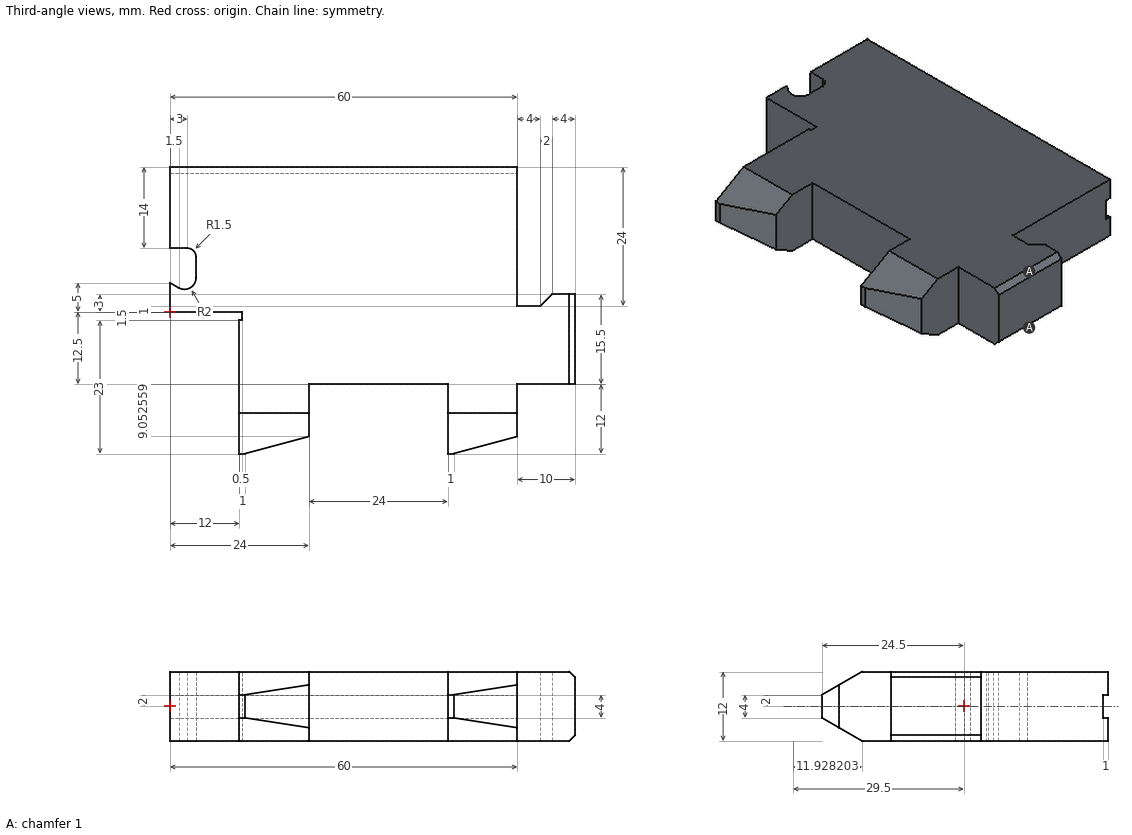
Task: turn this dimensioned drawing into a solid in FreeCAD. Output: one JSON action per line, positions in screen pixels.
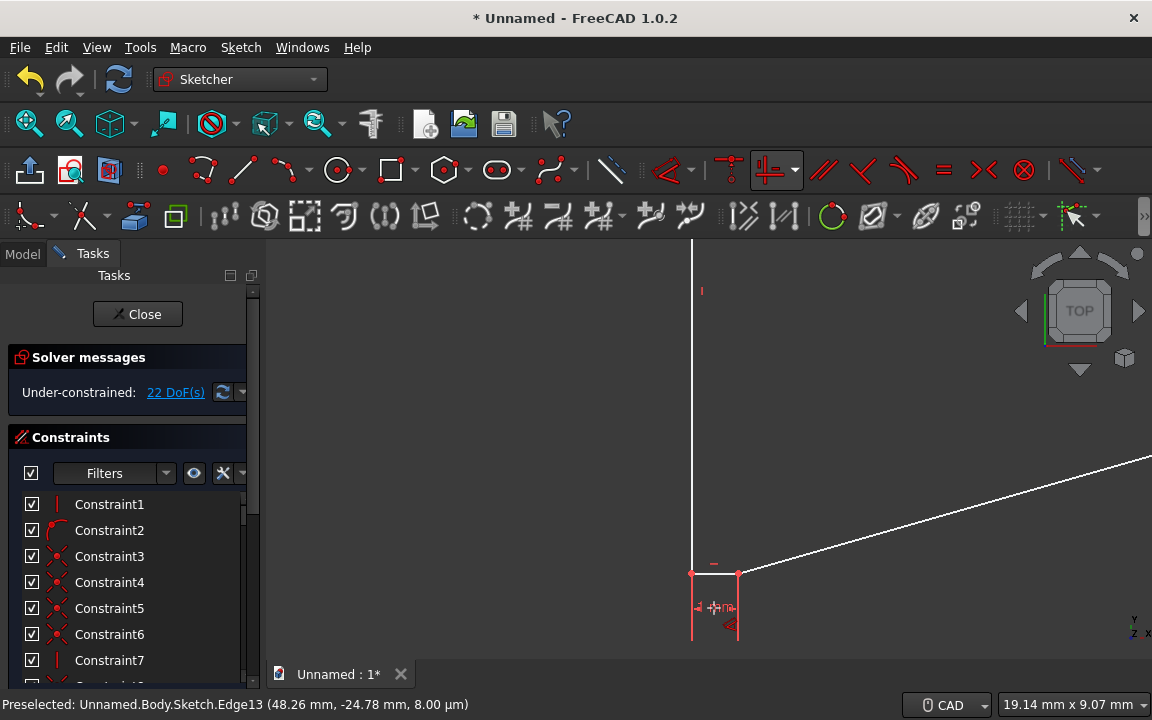
{"action": "scroll", "coordinate": [709, 578], "scroll_direction": "down", "scroll_amount": 11}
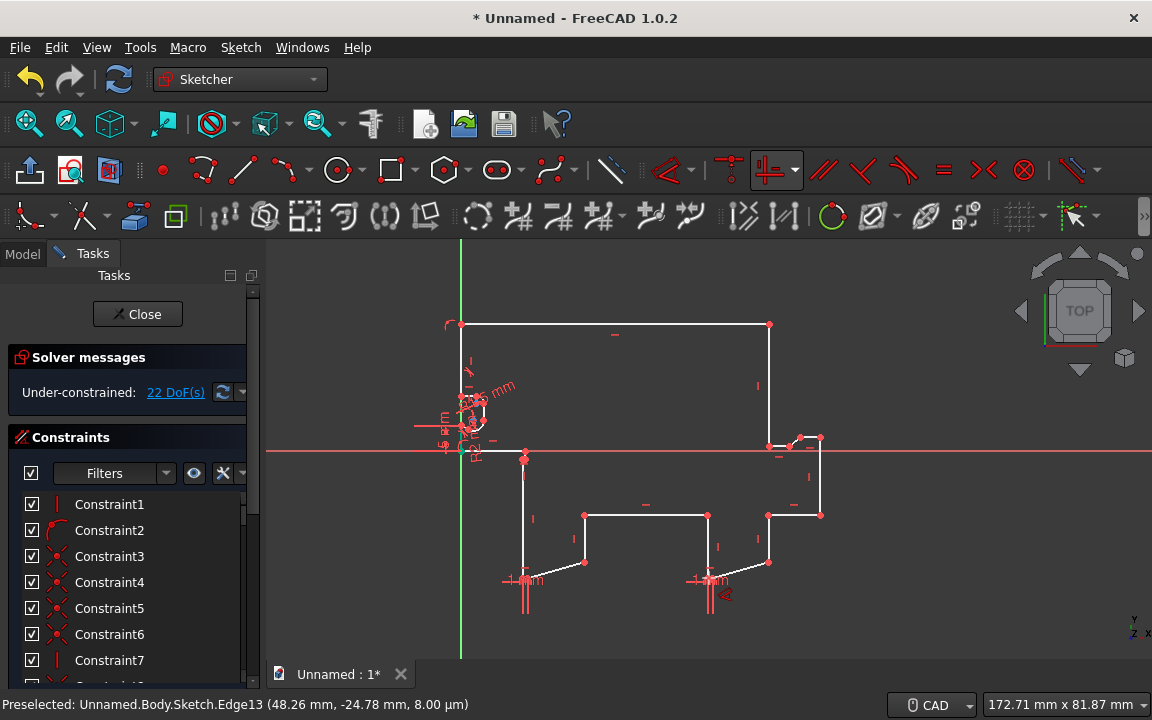
{"action": "scroll", "coordinate": [814, 437], "scroll_direction": "up", "scroll_amount": 5}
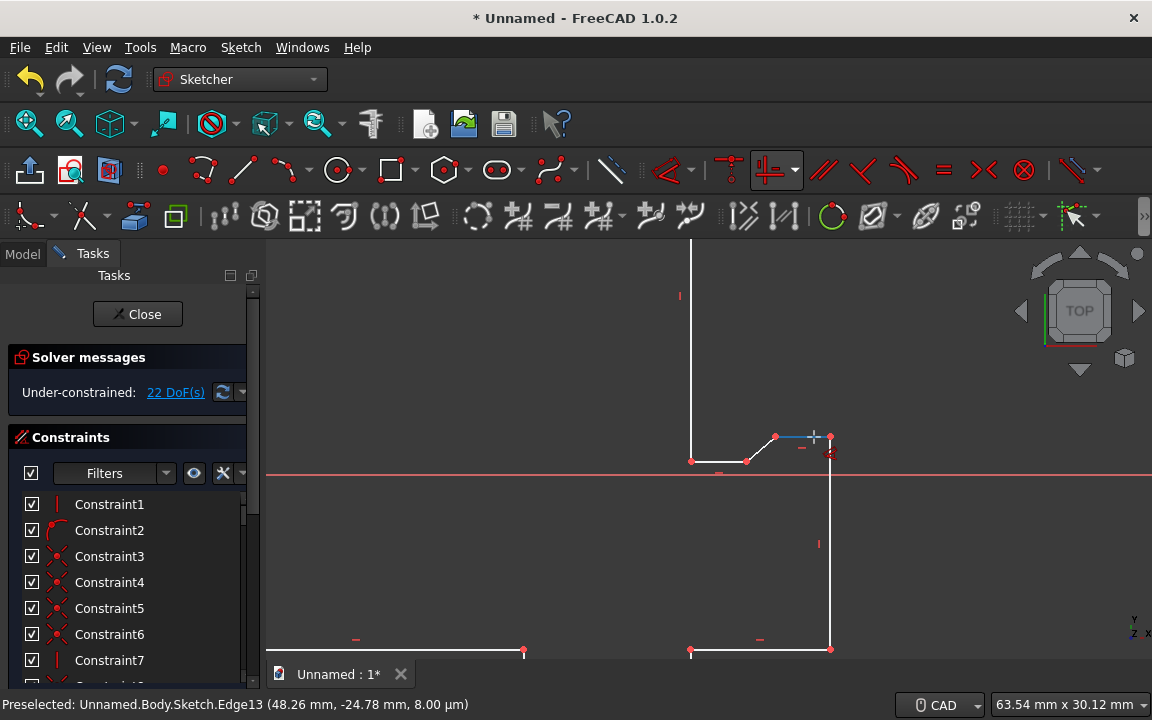
{"action": "left_click", "coordinate": [814, 437]}
{"action": "left_click", "coordinate": [803, 403]}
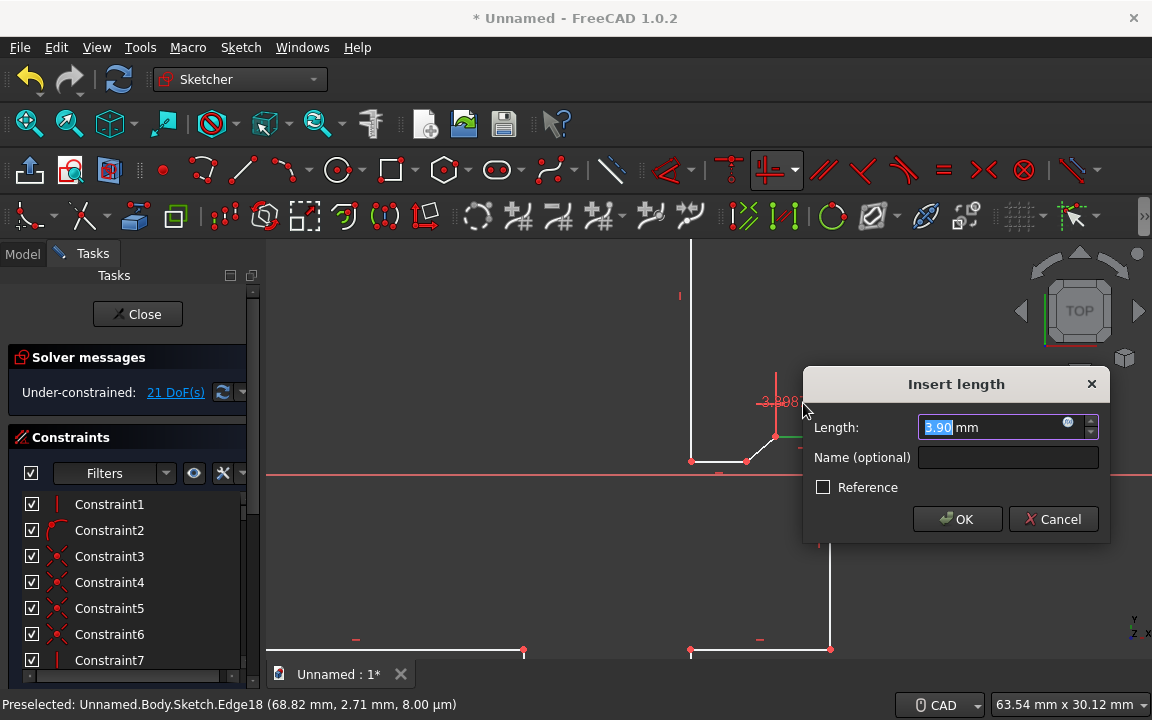
{"action": "type", "text": "4"}
{"action": "key", "text": "Return"}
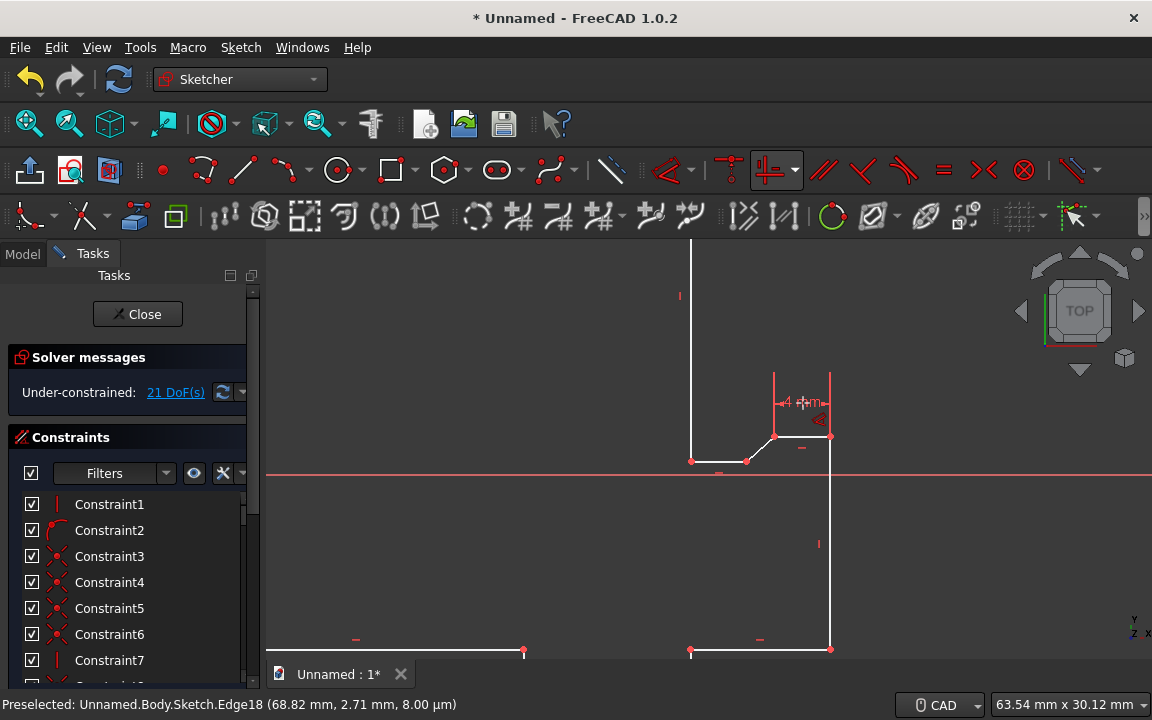
{"action": "left_click", "coordinate": [730, 462]}
{"action": "left_click", "coordinate": [719, 428]}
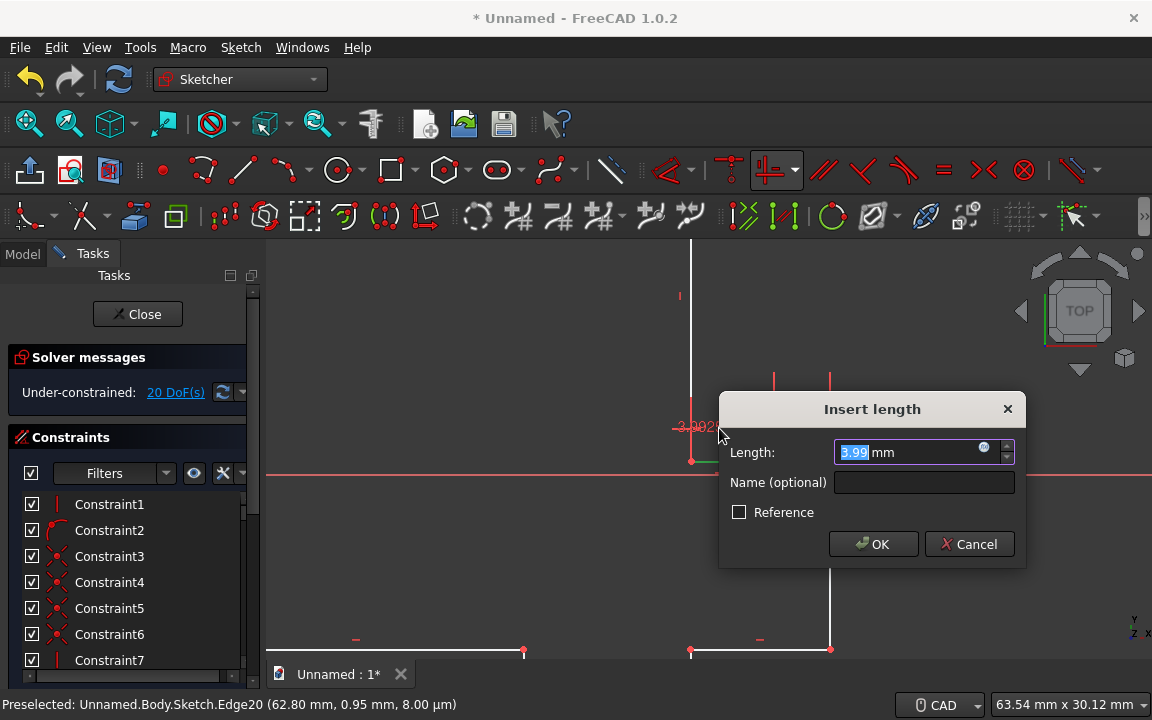
{"action": "type", "text": "4"}
{"action": "key", "text": "Return"}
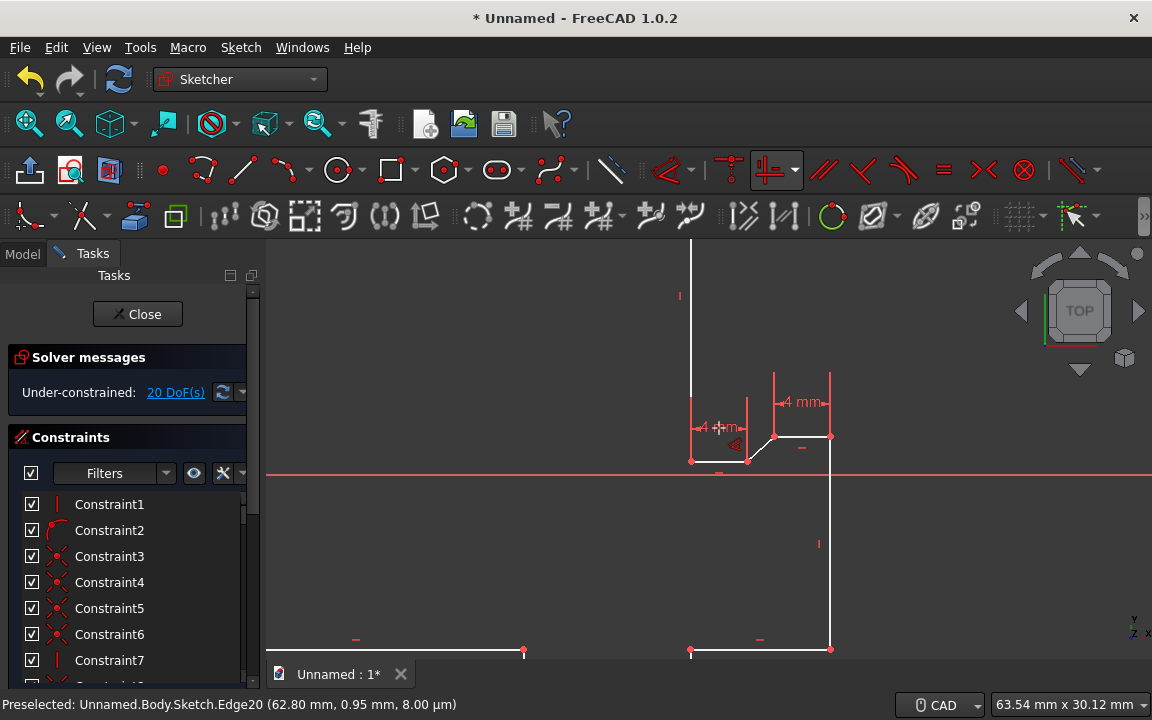
{"action": "scroll", "coordinate": [814, 436], "scroll_direction": "down", "scroll_amount": 5}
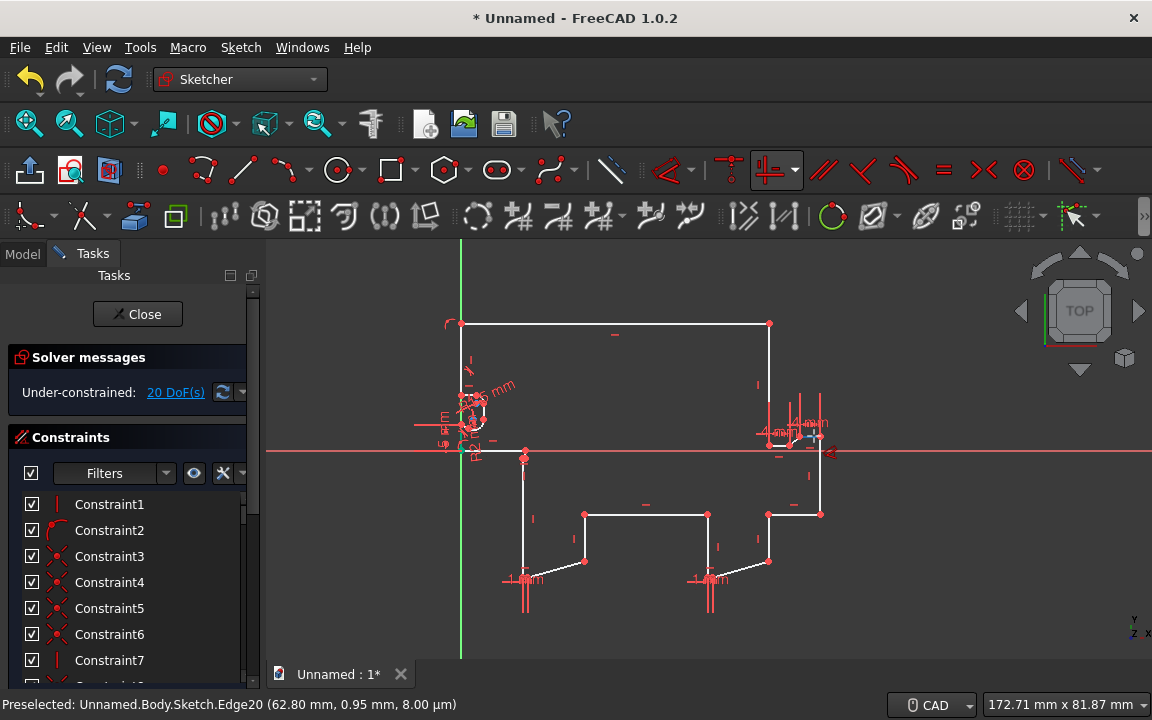
{"action": "scroll", "coordinate": [466, 395], "scroll_direction": "up", "scroll_amount": 6}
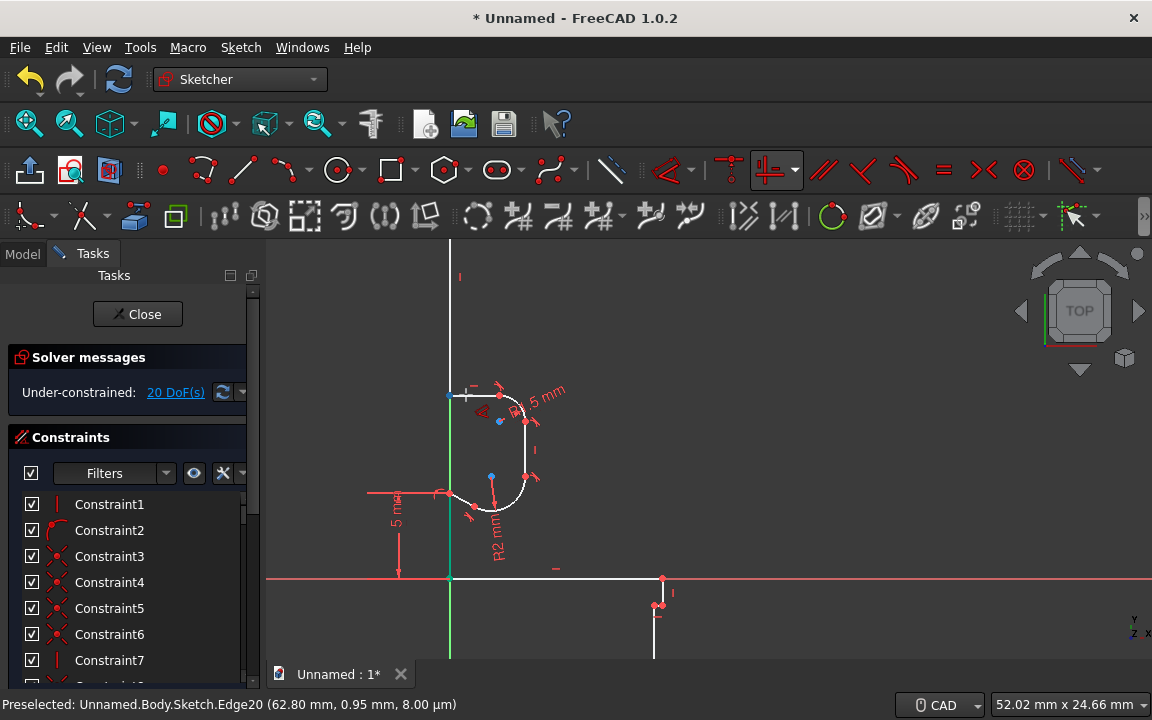
{"action": "left_click", "coordinate": [465, 396]}
{"action": "left_click", "coordinate": [475, 362]}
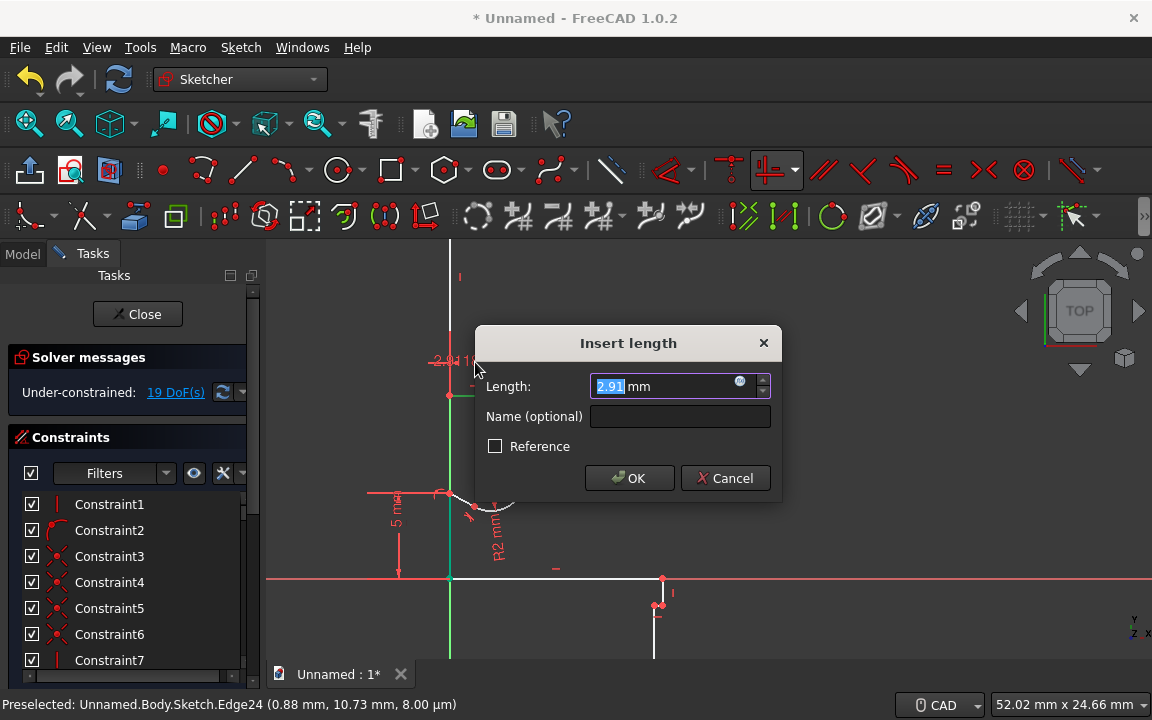
{"action": "type", "text": "3"}
{"action": "key", "text": "Return"}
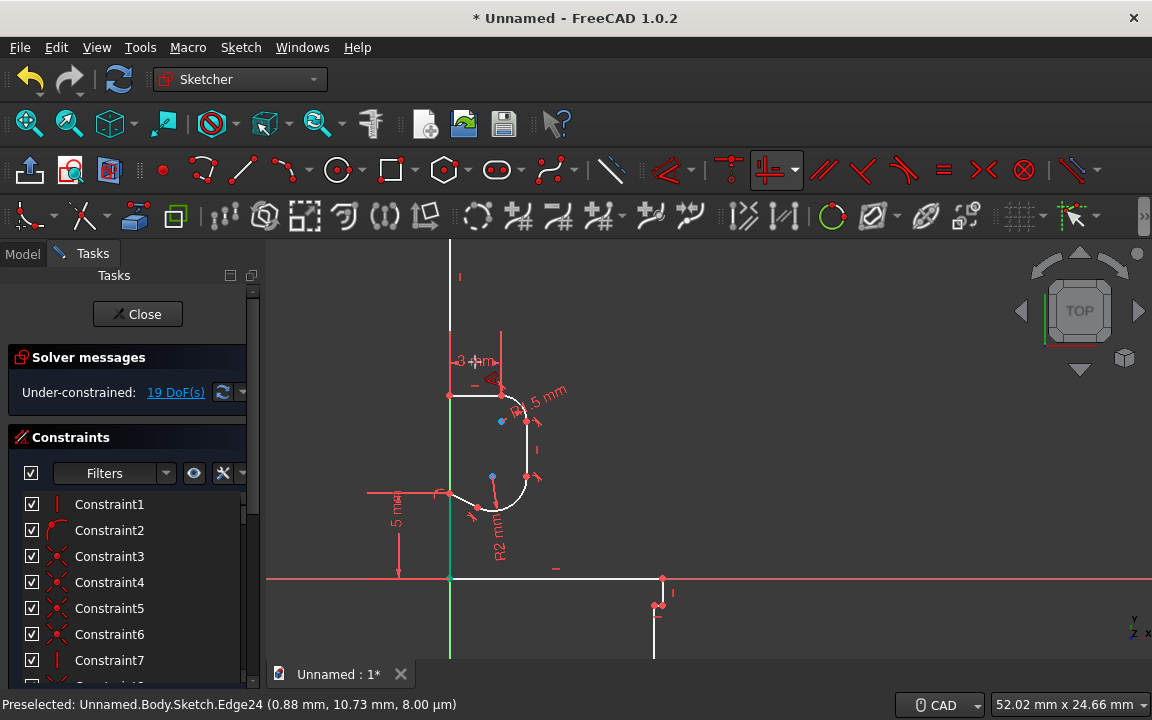
{"action": "scroll", "coordinate": [466, 395], "scroll_direction": "down", "scroll_amount": 6}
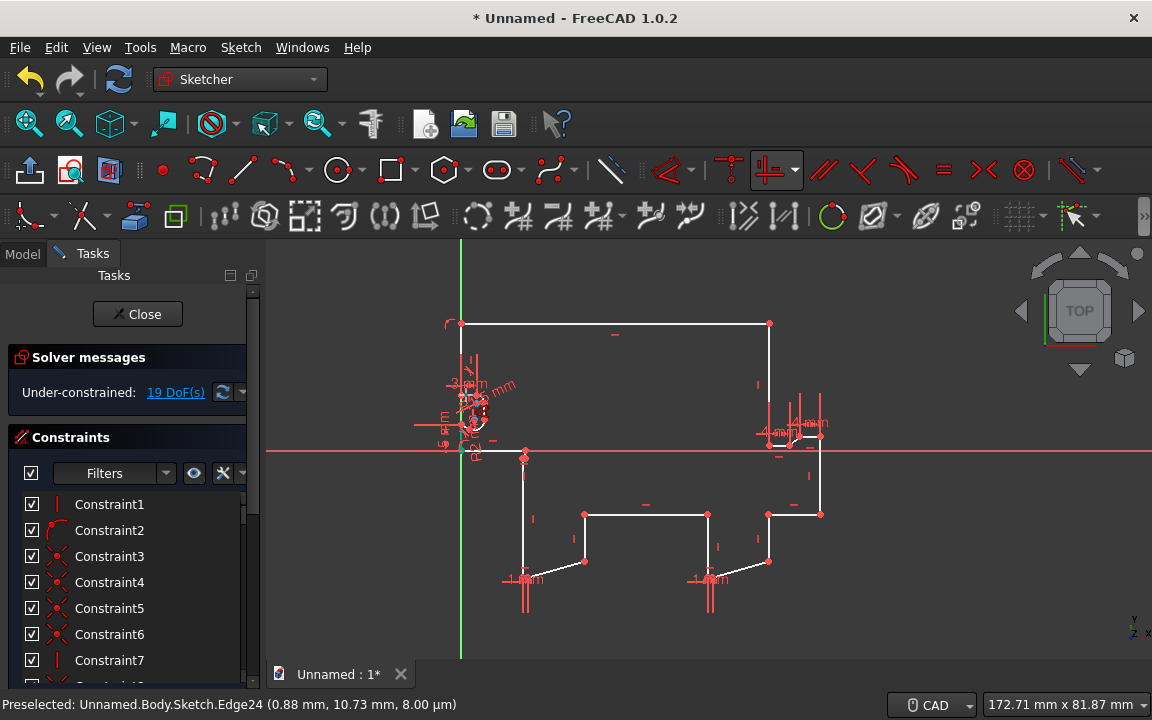
{"action": "left_click", "coordinate": [523, 494]}
{"action": "left_click", "coordinate": [489, 518]}